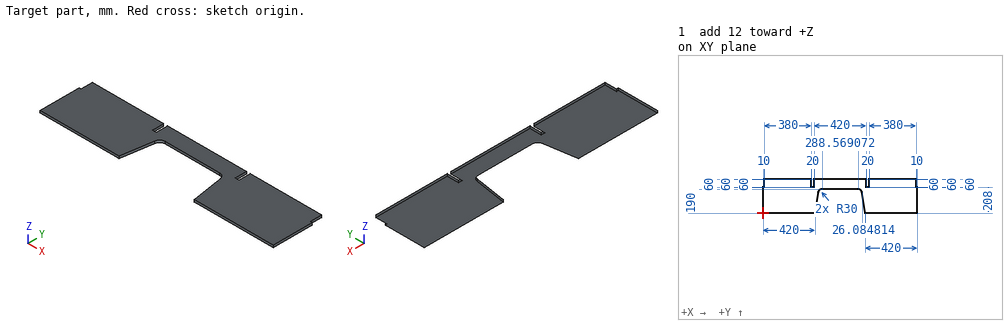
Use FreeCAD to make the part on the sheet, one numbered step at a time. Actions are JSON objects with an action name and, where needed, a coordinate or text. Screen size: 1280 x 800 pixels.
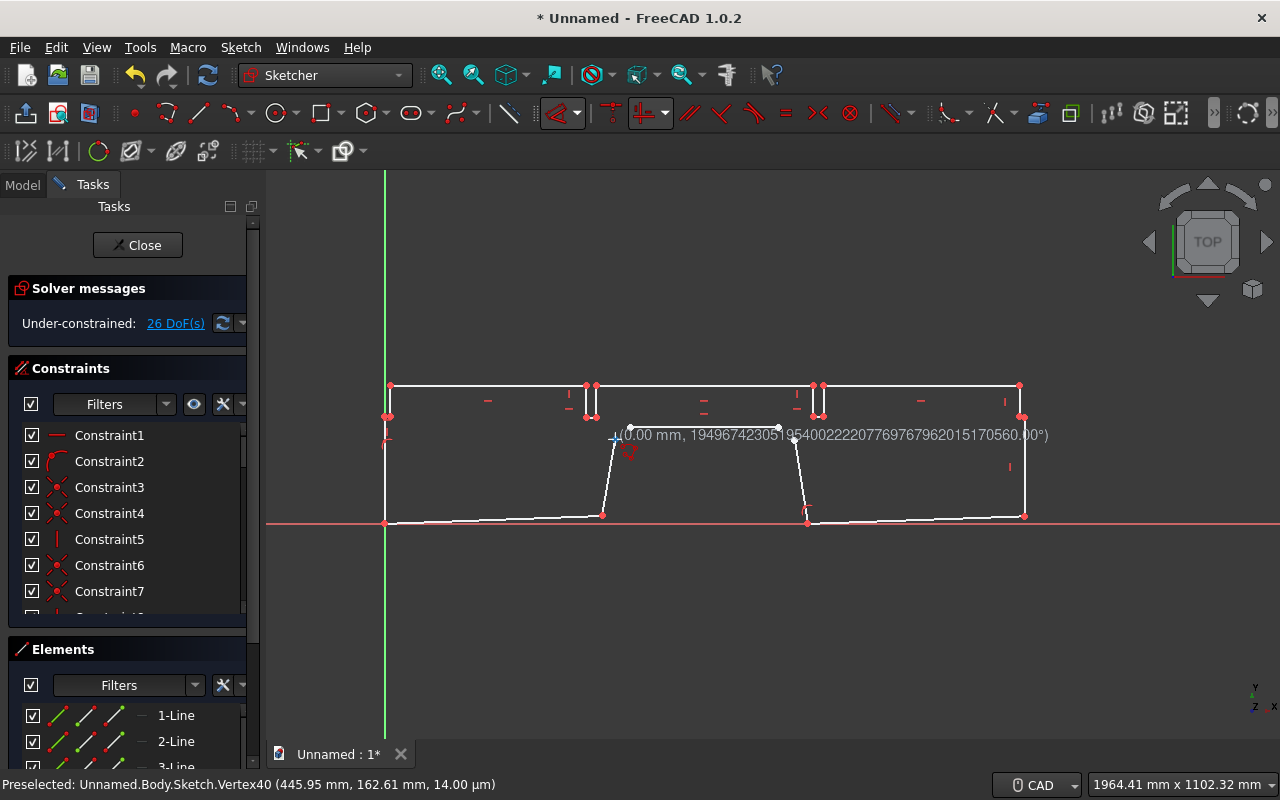
{"action": "key", "text": "g 3 a"}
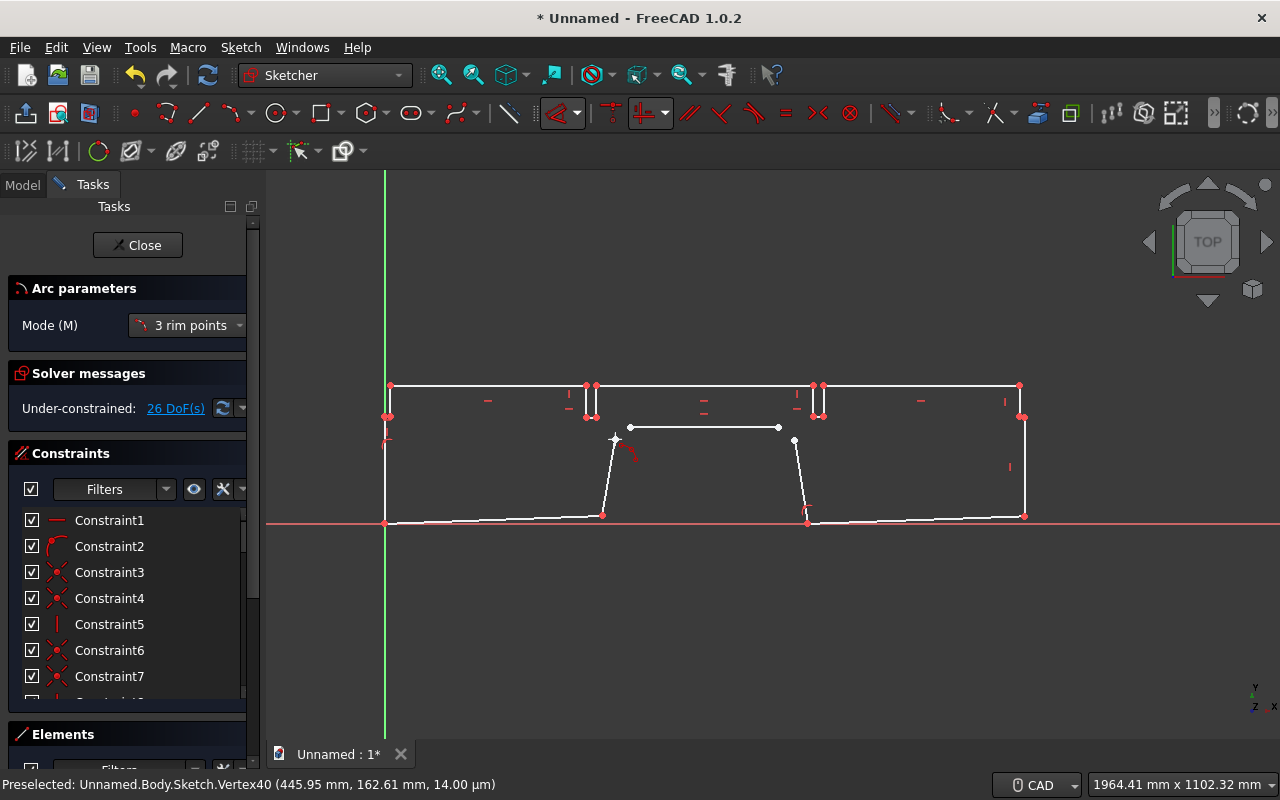
{"action": "left_click", "coordinate": [779, 427]}
{"action": "left_click", "coordinate": [795, 440]}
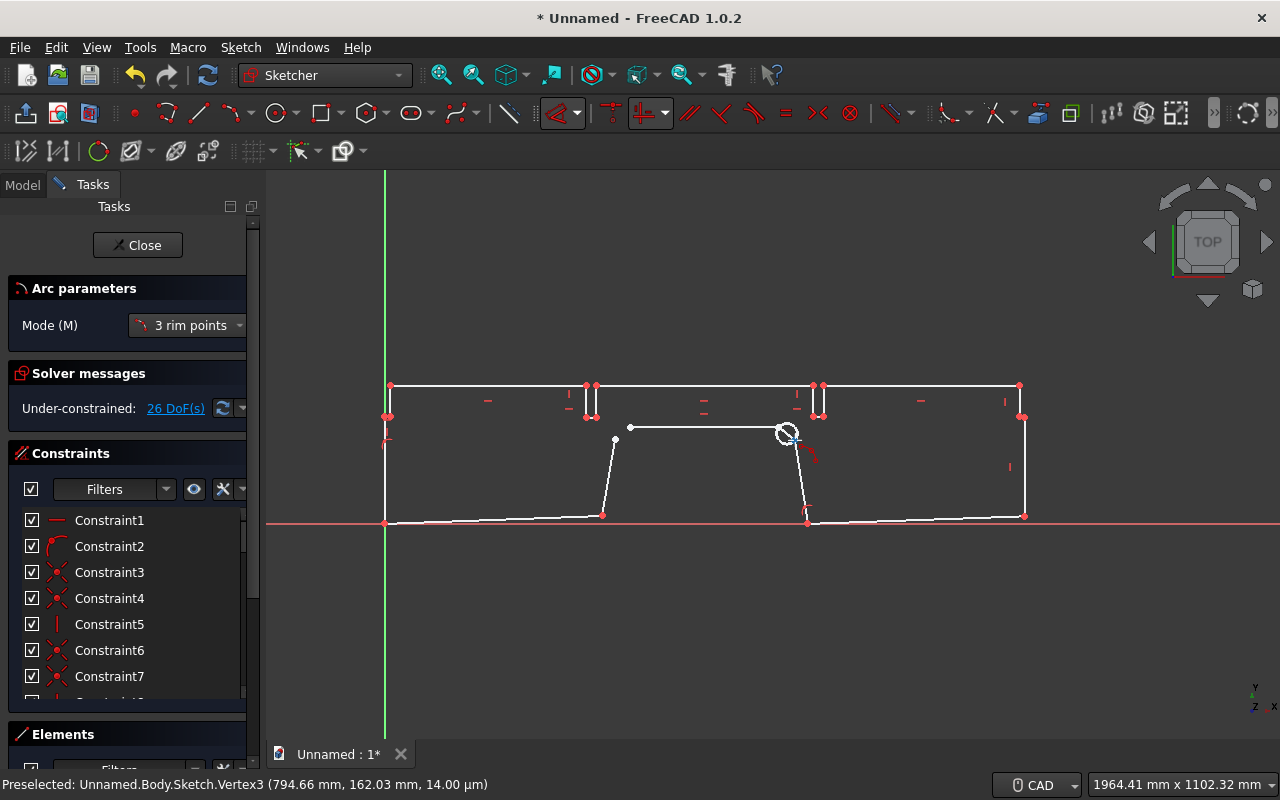
{"action": "scroll", "coordinate": [789, 430], "scroll_direction": "up", "scroll_amount": 8}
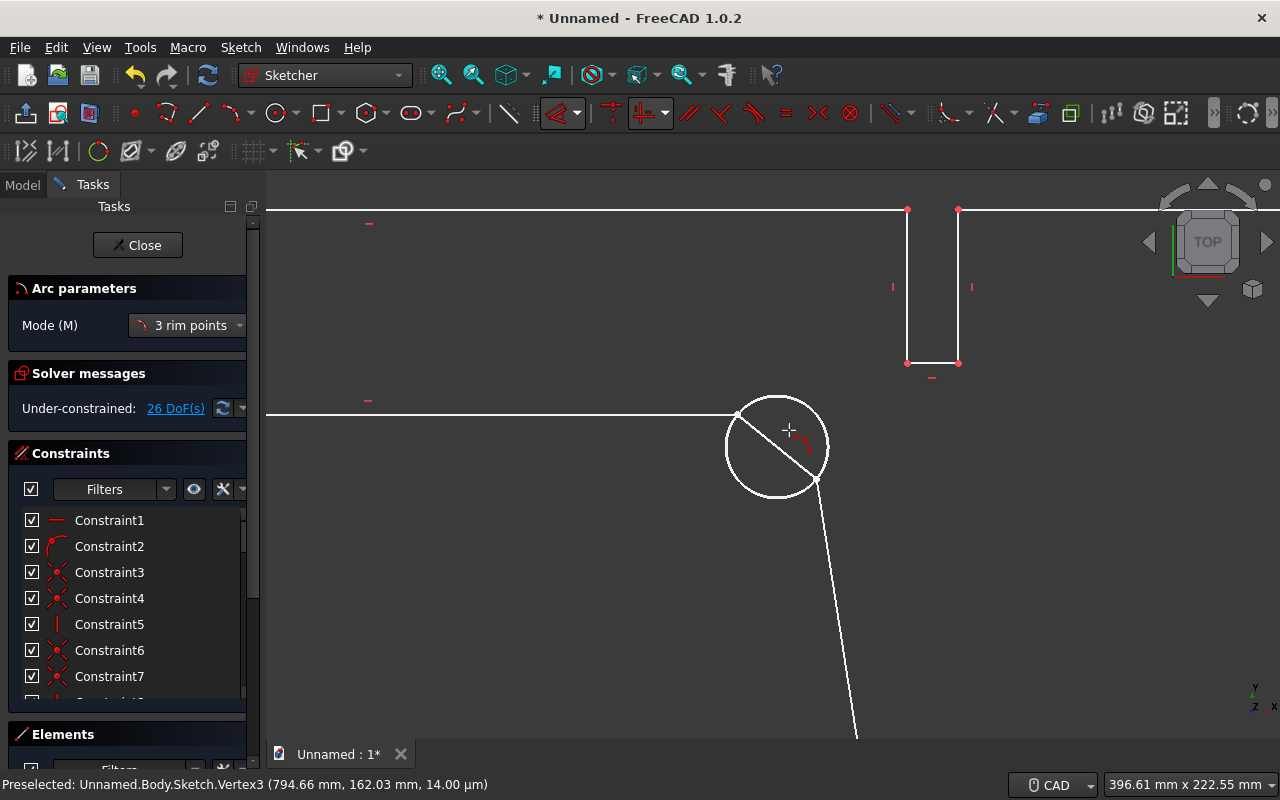
{"action": "left_click", "coordinate": [789, 426]}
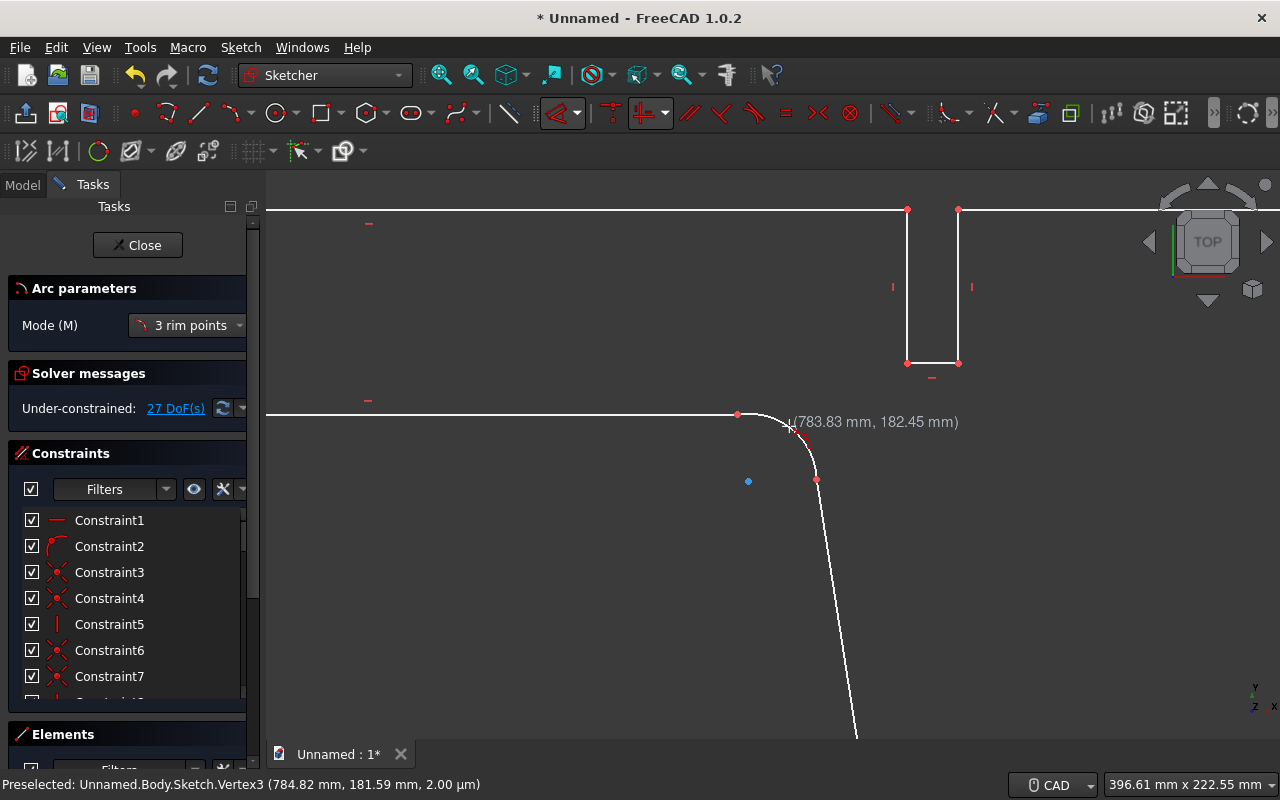
{"action": "scroll", "coordinate": [789, 430], "scroll_direction": "down", "scroll_amount": 8}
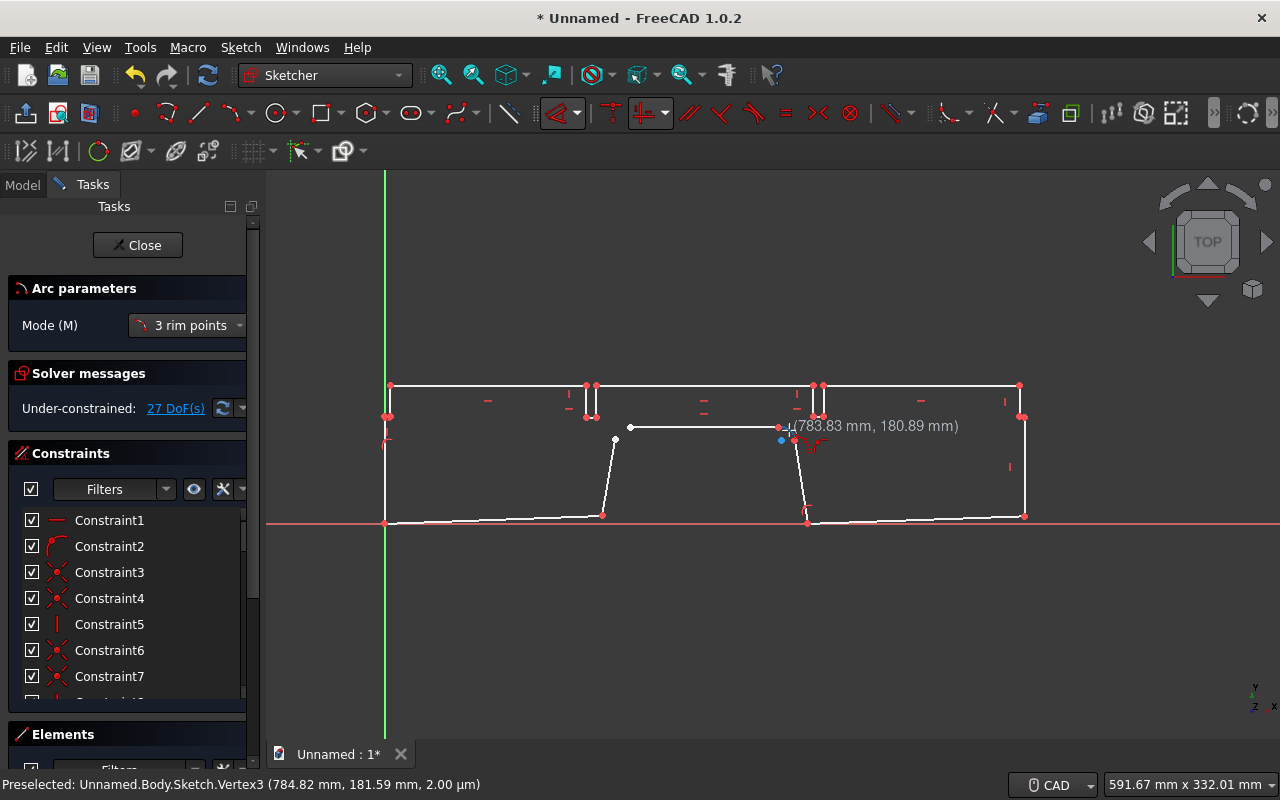
{"action": "left_click", "coordinate": [615, 440]}
{"action": "left_click", "coordinate": [630, 427]}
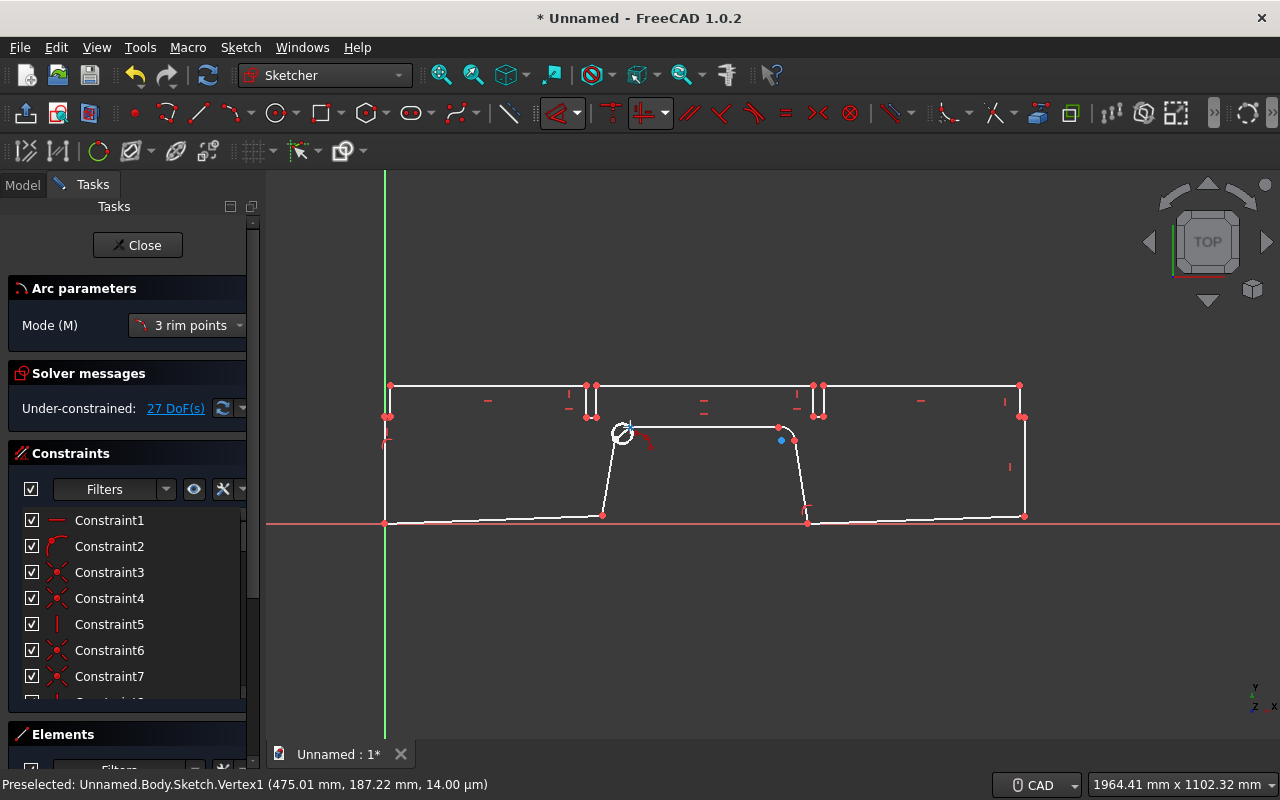
{"action": "scroll", "coordinate": [620, 430], "scroll_direction": "up", "scroll_amount": 8}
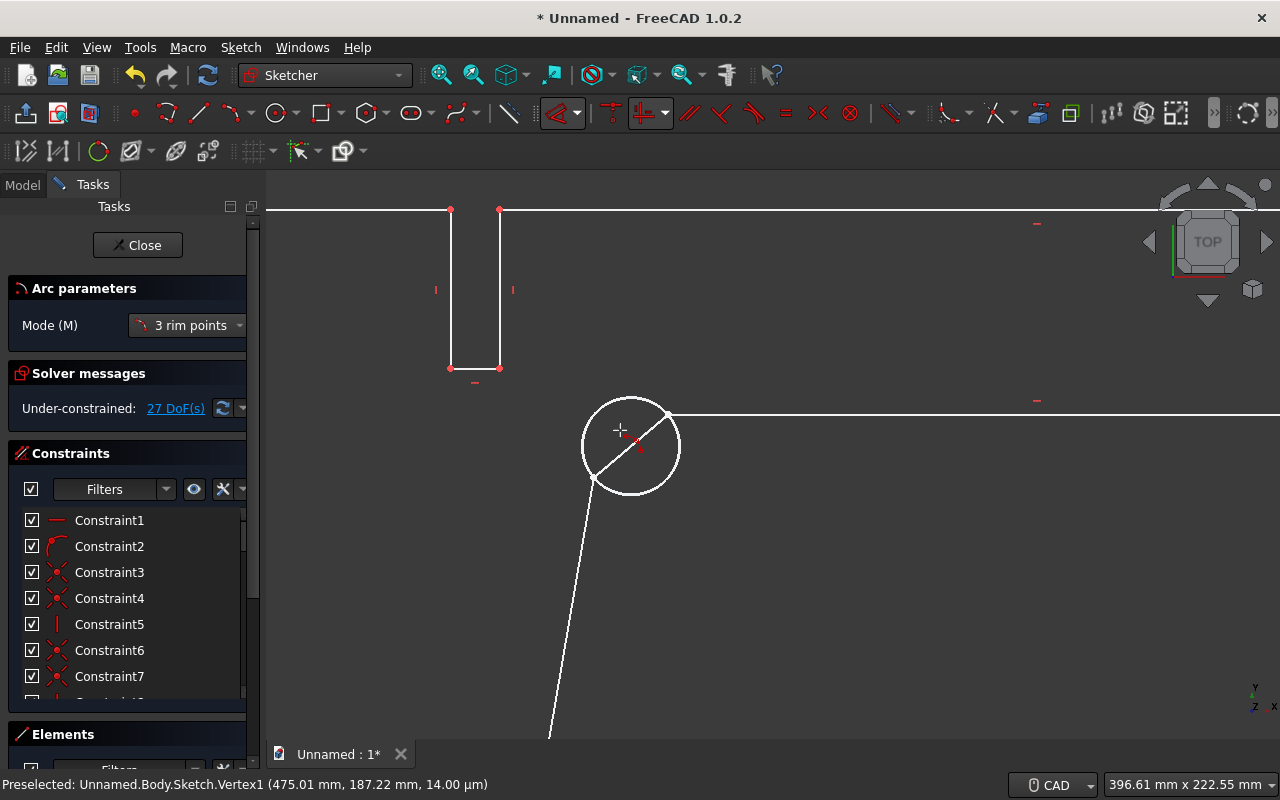
{"action": "left_click", "coordinate": [620, 426]}
{"action": "key", "text": "Escape"}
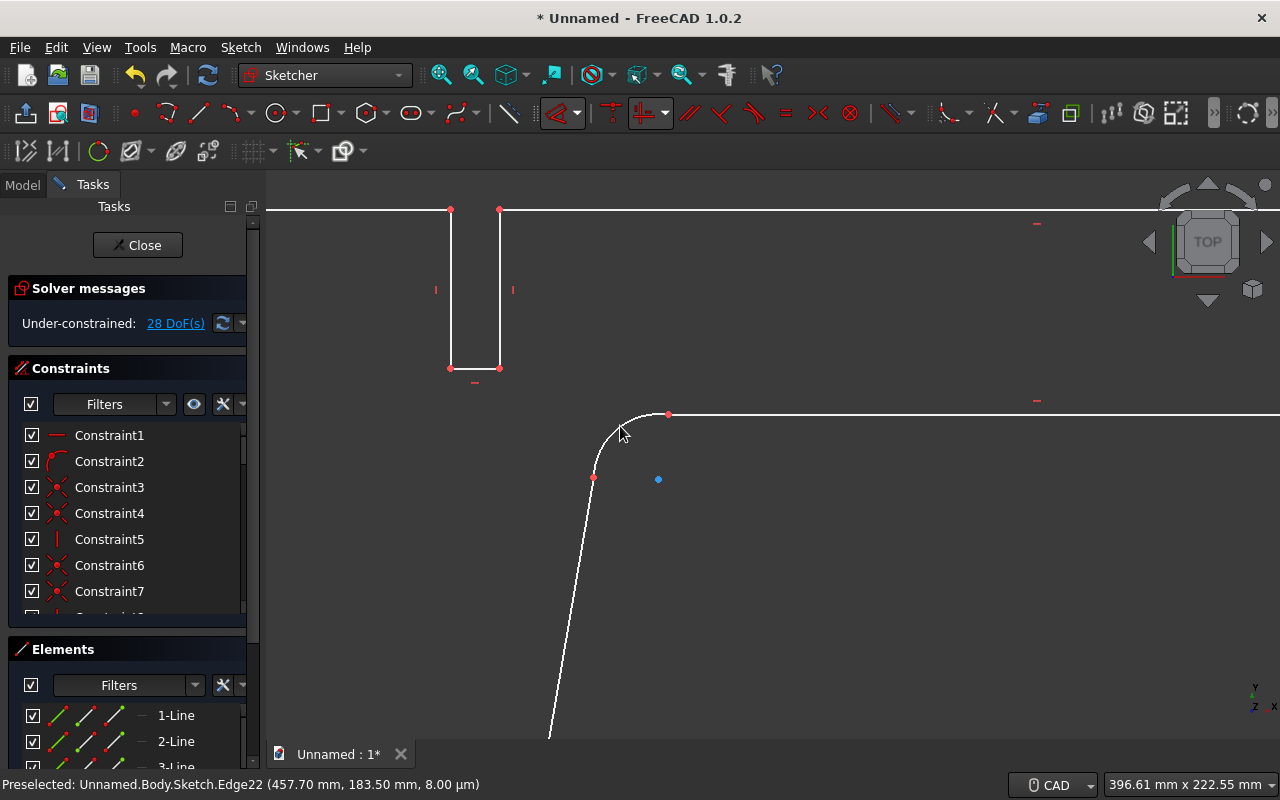
{"action": "scroll", "coordinate": [620, 430], "scroll_direction": "down", "scroll_amount": 8}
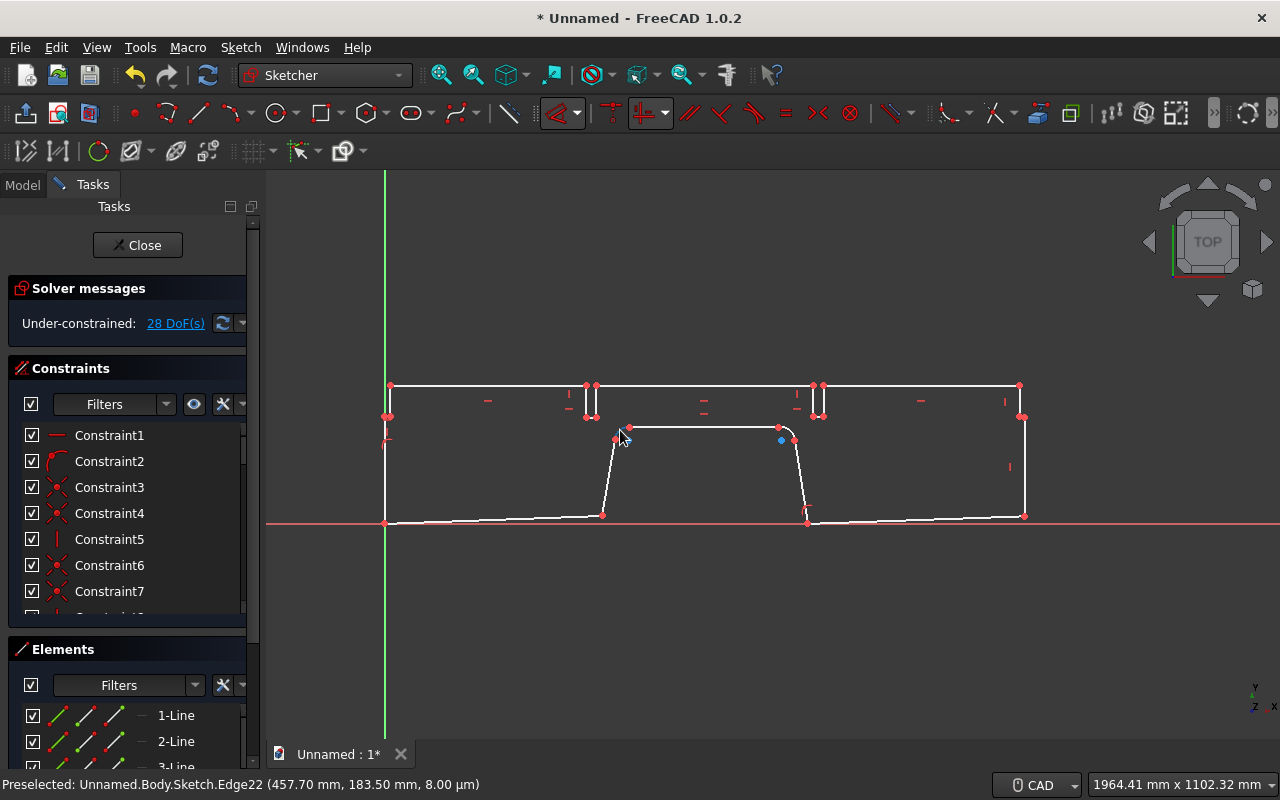
{"action": "left_click", "coordinate": [675, 427]}